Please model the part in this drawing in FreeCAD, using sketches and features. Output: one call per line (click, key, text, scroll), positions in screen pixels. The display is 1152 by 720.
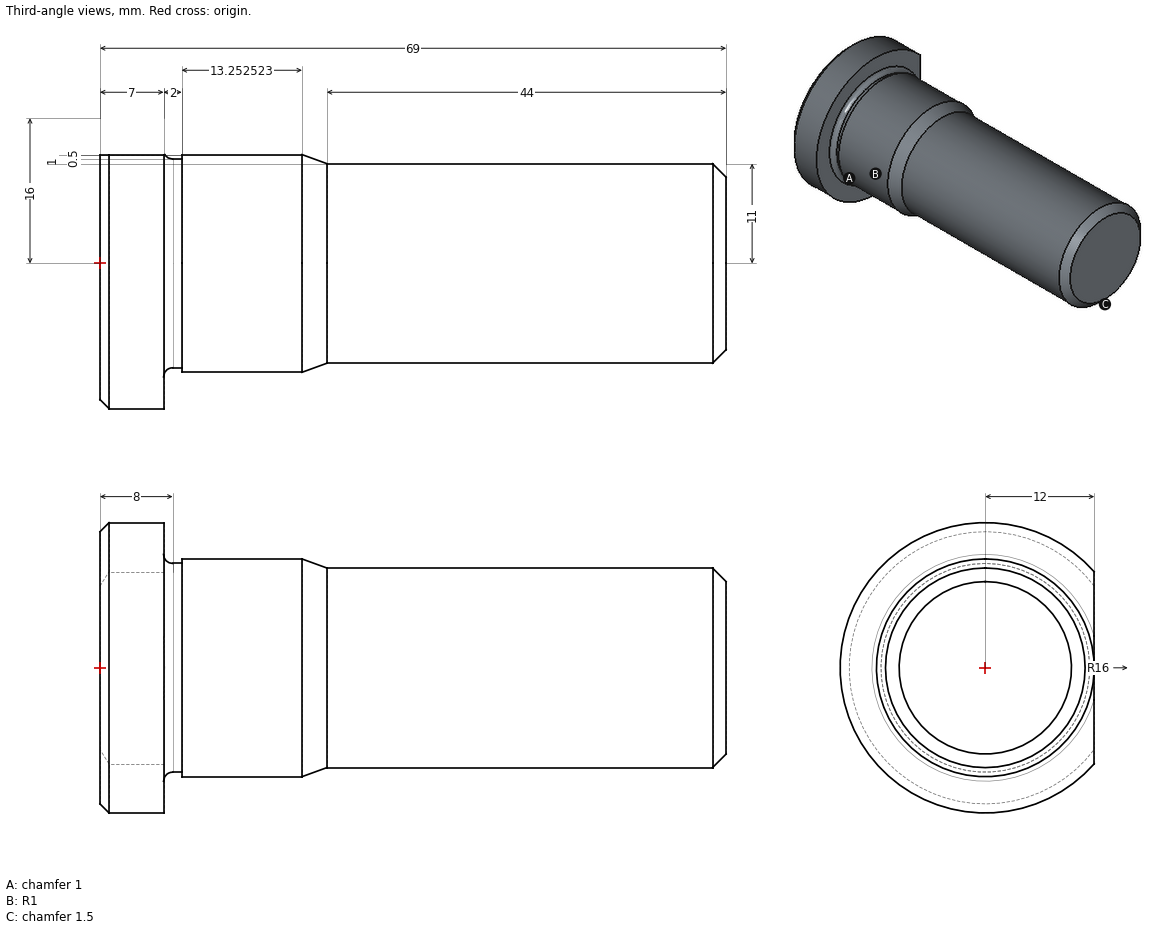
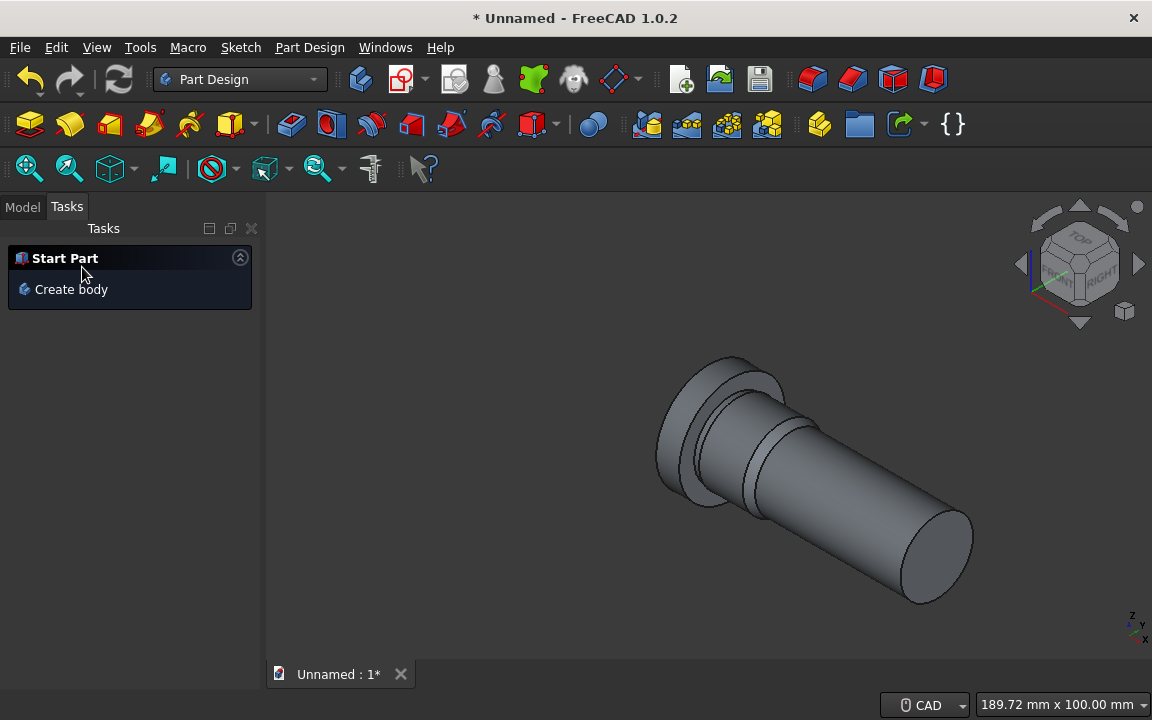
click(725, 357)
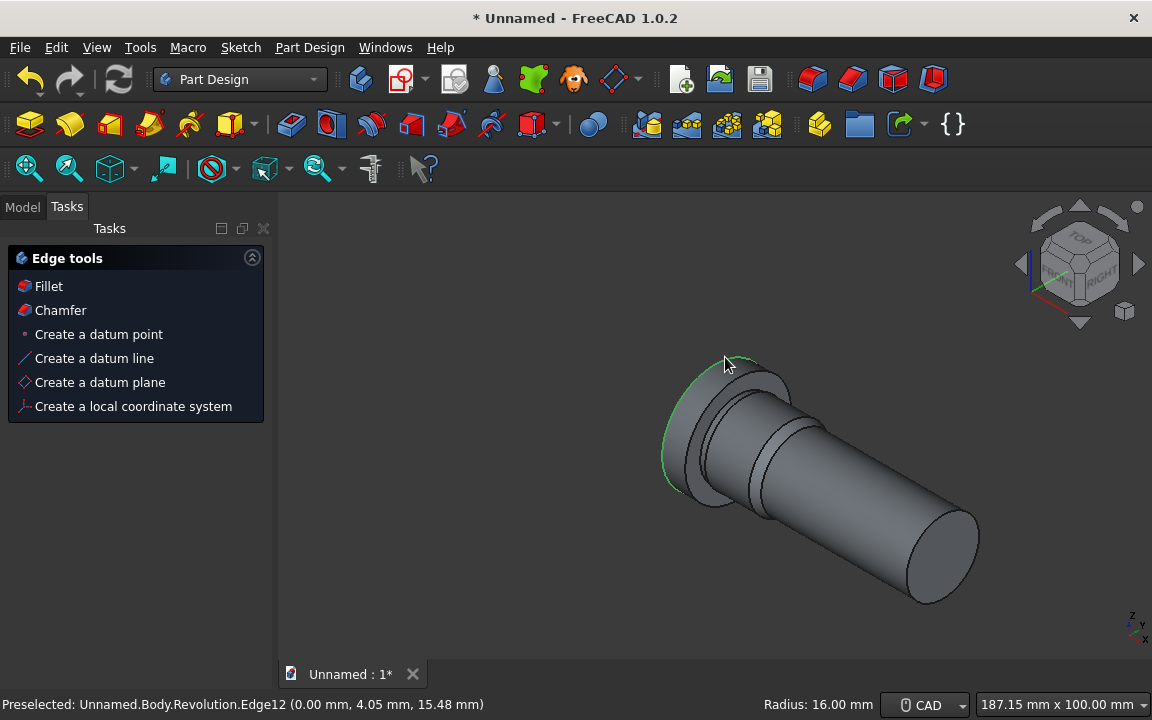
click(854, 80)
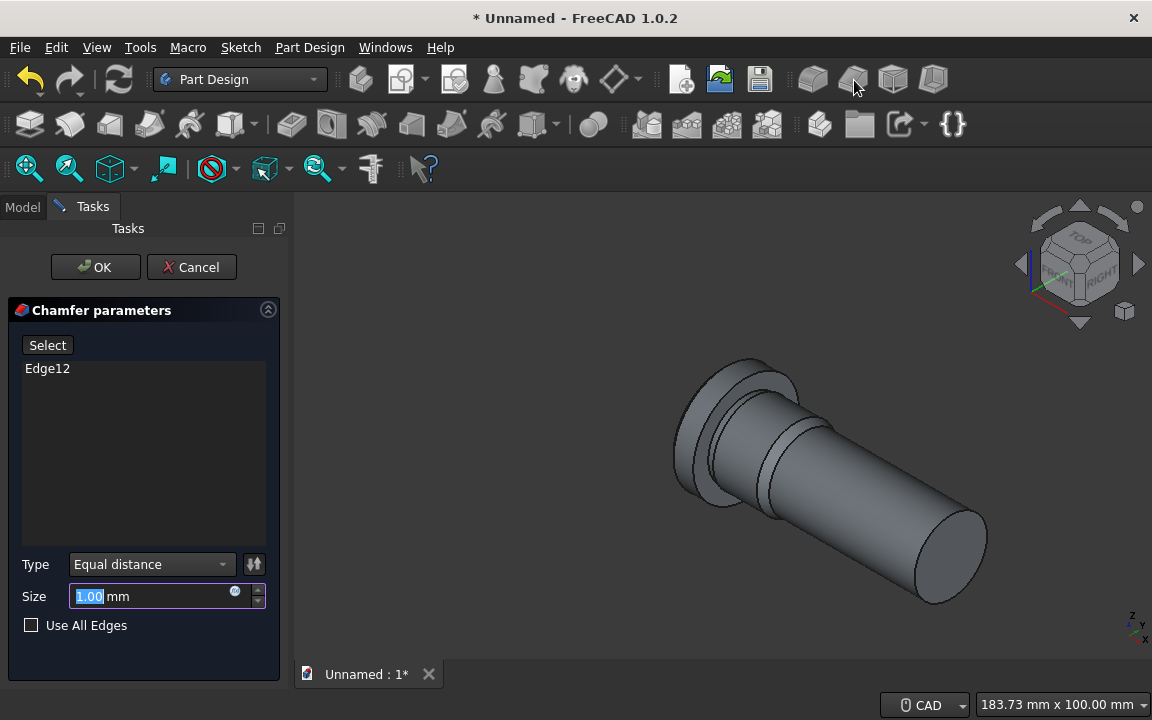
text(1)
key(Tab)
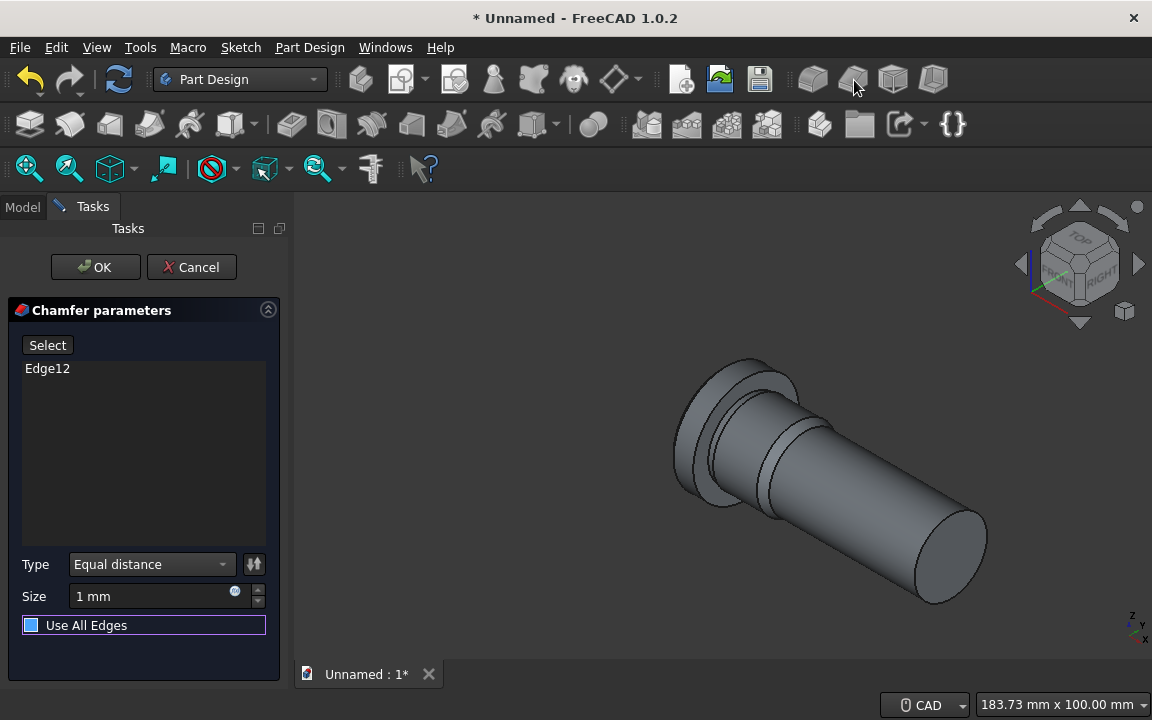
click(96, 267)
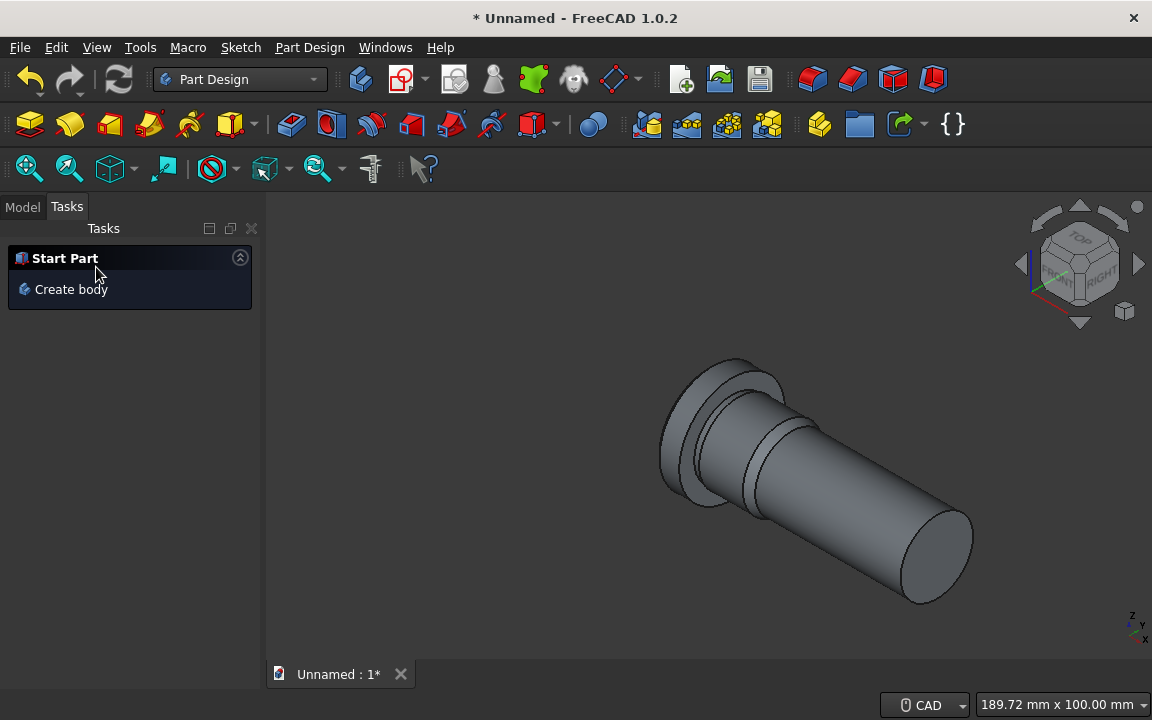
key(2)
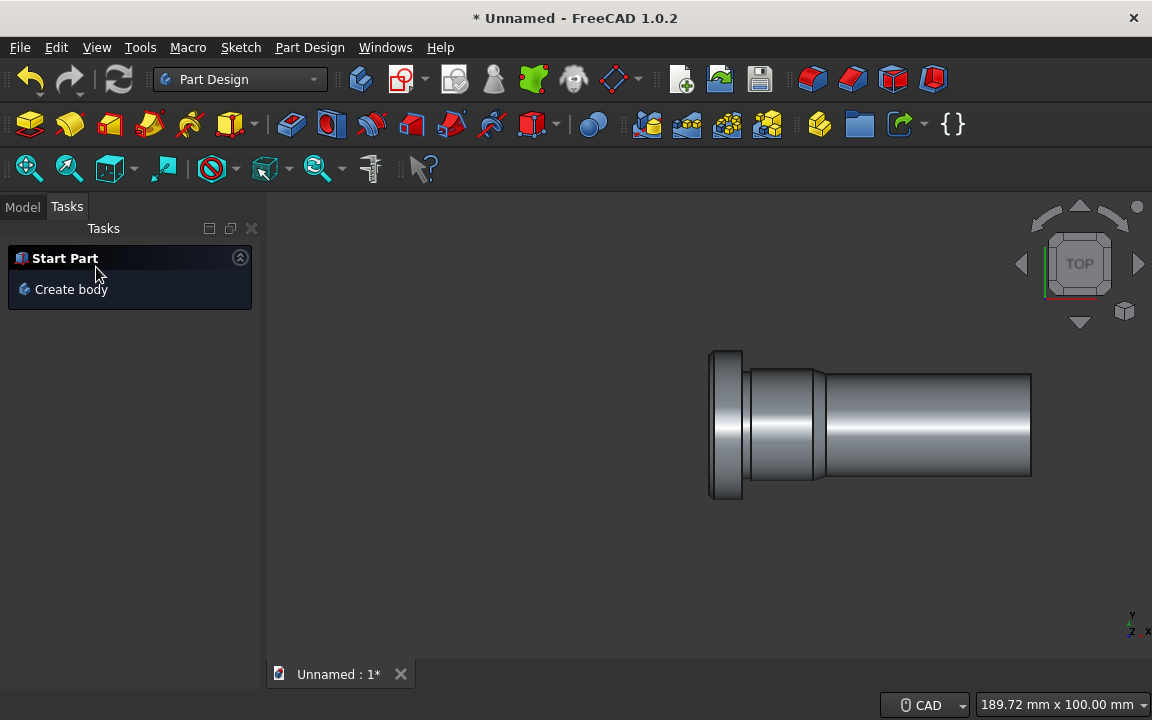
click(30, 170)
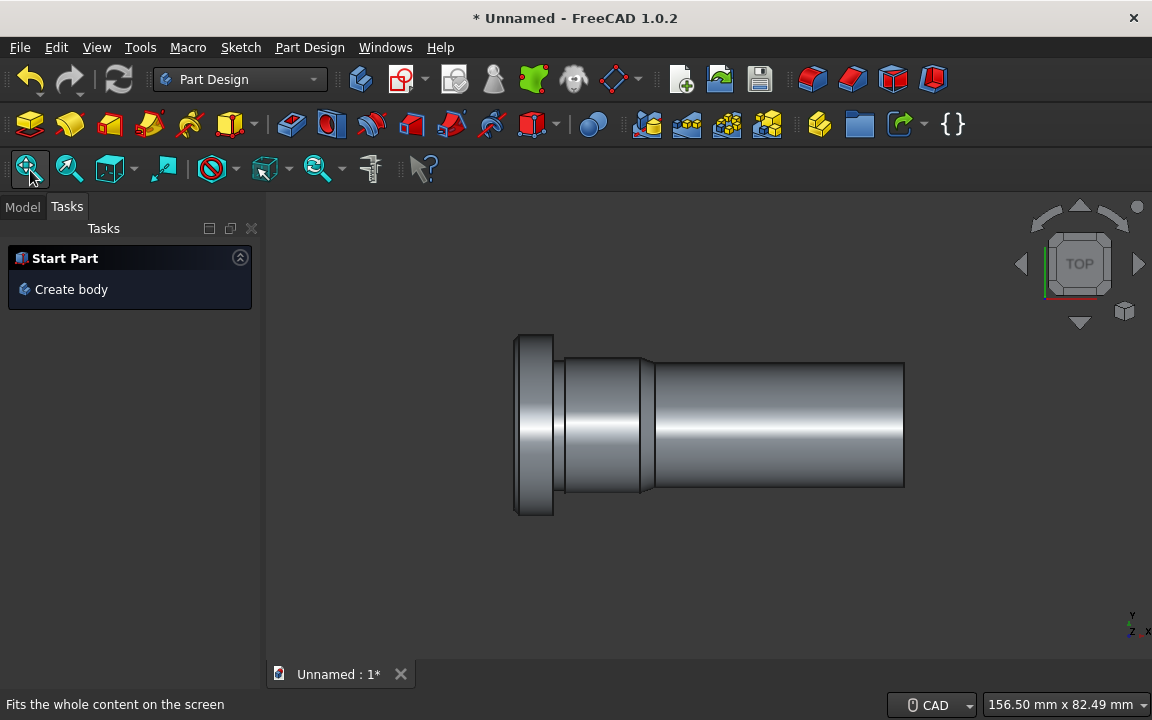
key(0)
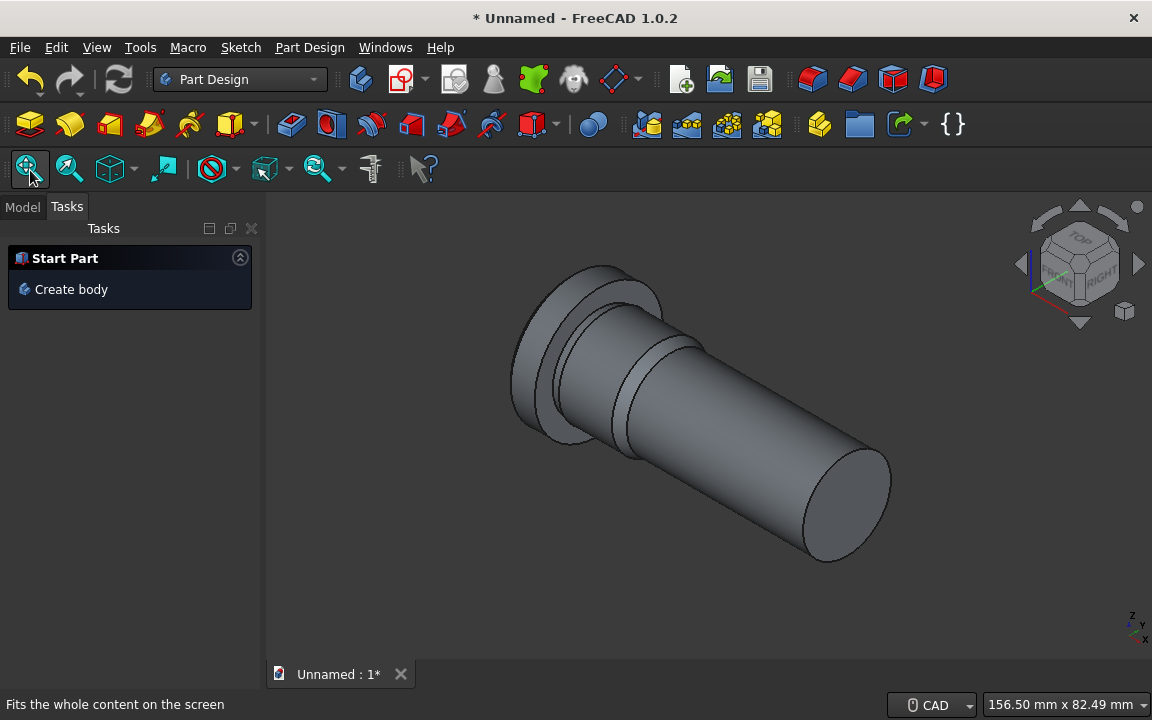
key(1)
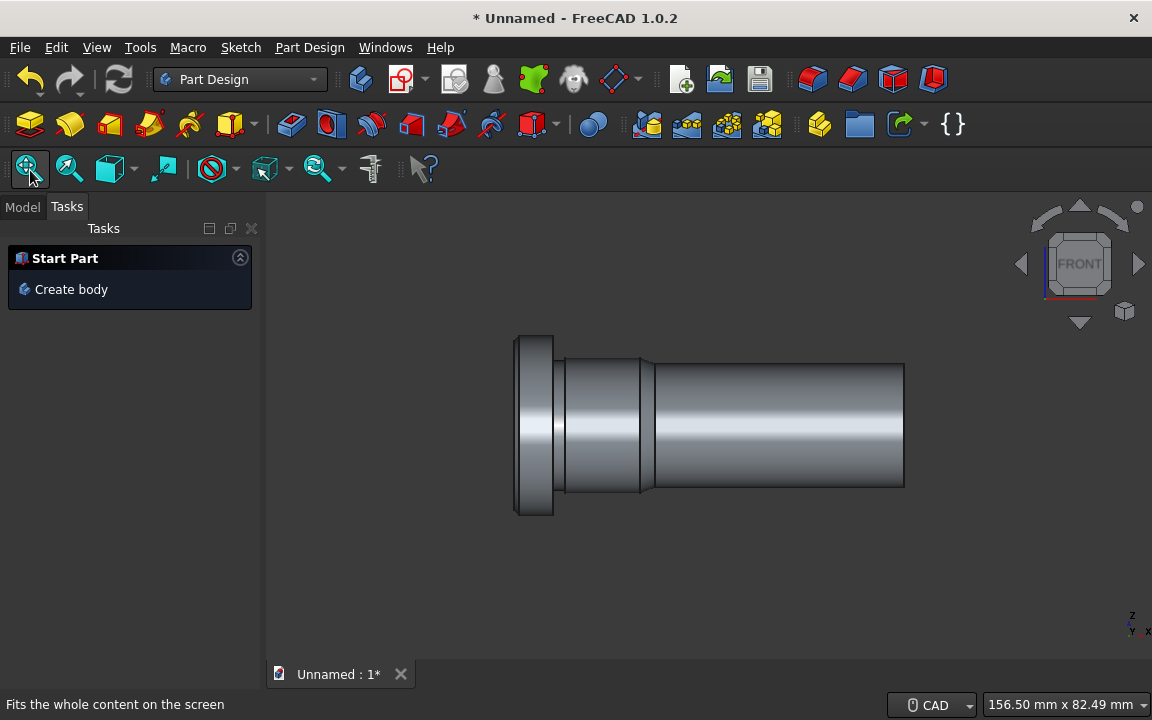
click(30, 170)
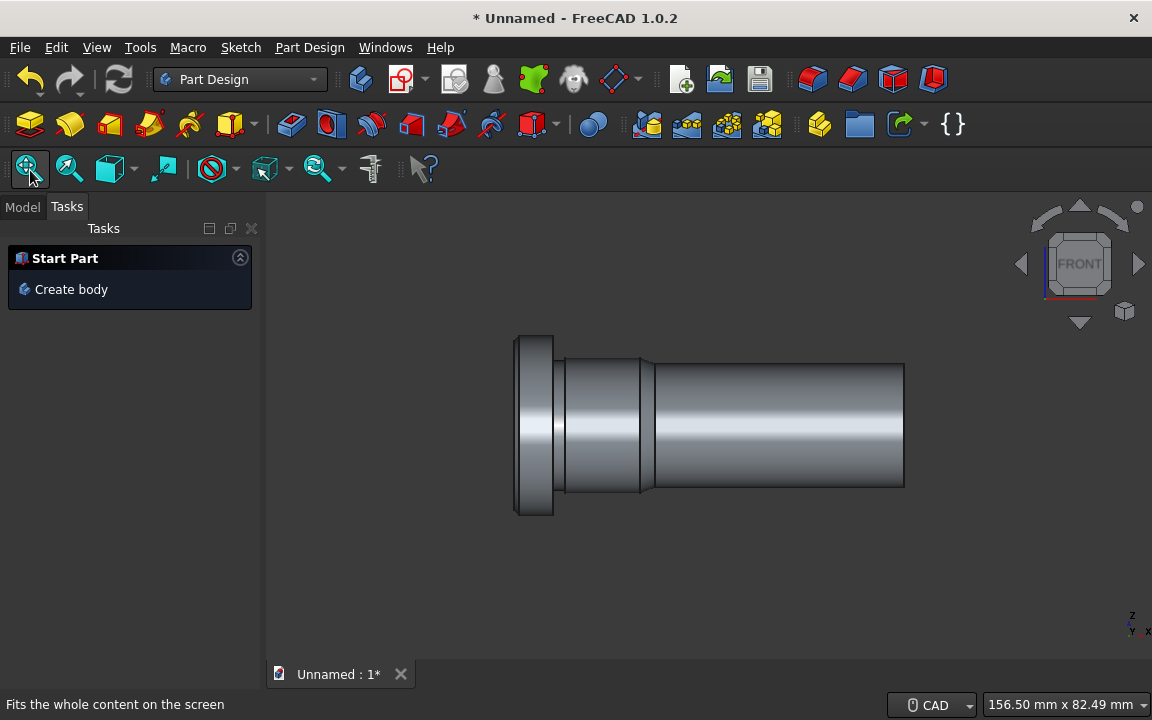
key(3)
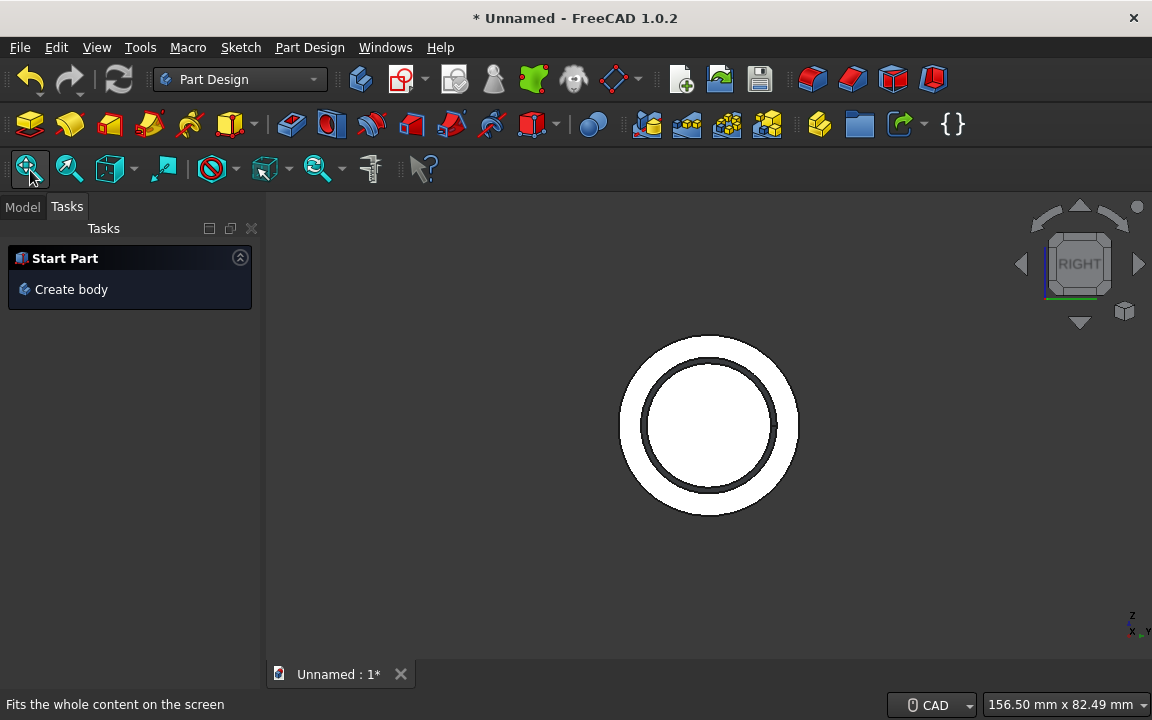
click(30, 170)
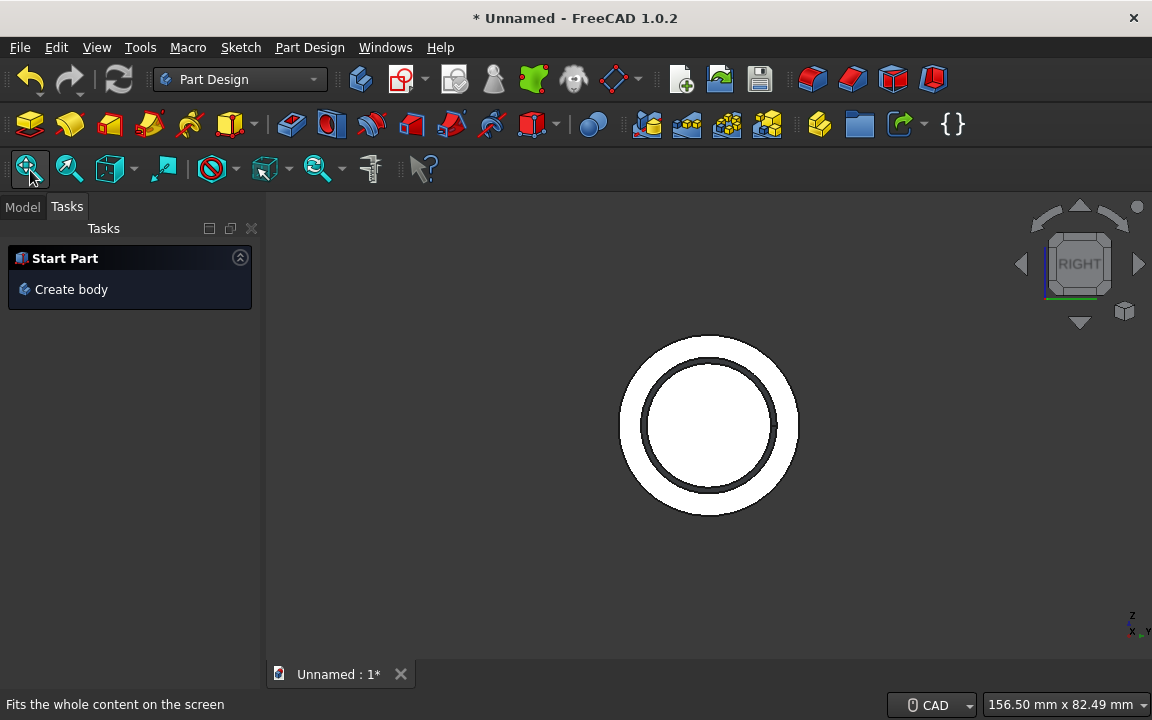
key(5)